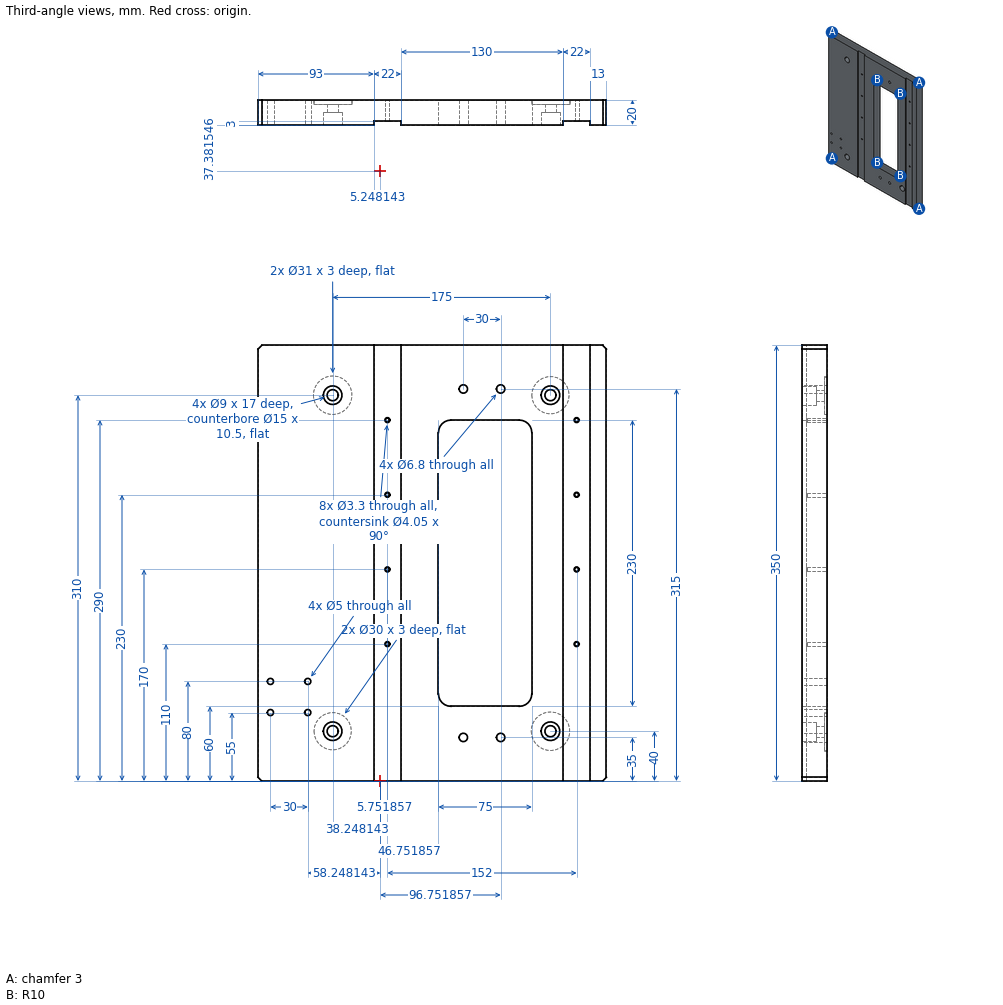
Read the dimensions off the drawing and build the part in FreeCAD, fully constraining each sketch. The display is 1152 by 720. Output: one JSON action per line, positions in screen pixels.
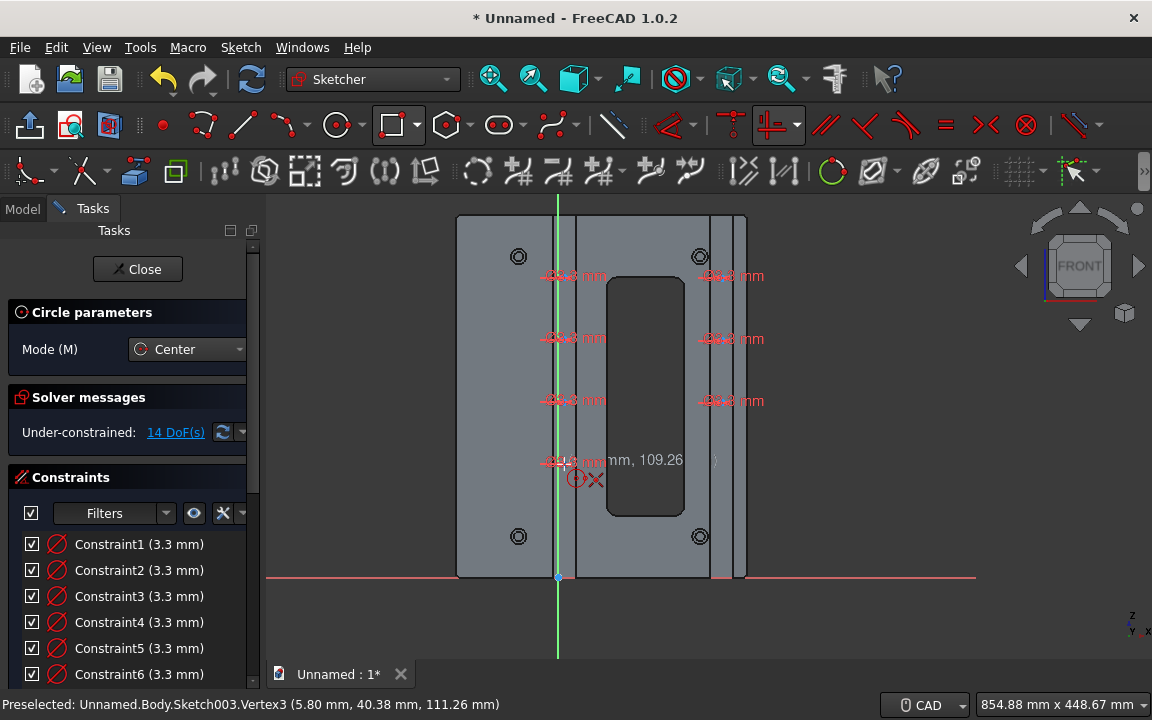
{"action": "scroll", "coordinate": [722, 464], "scroll_direction": "up", "scroll_amount": 13}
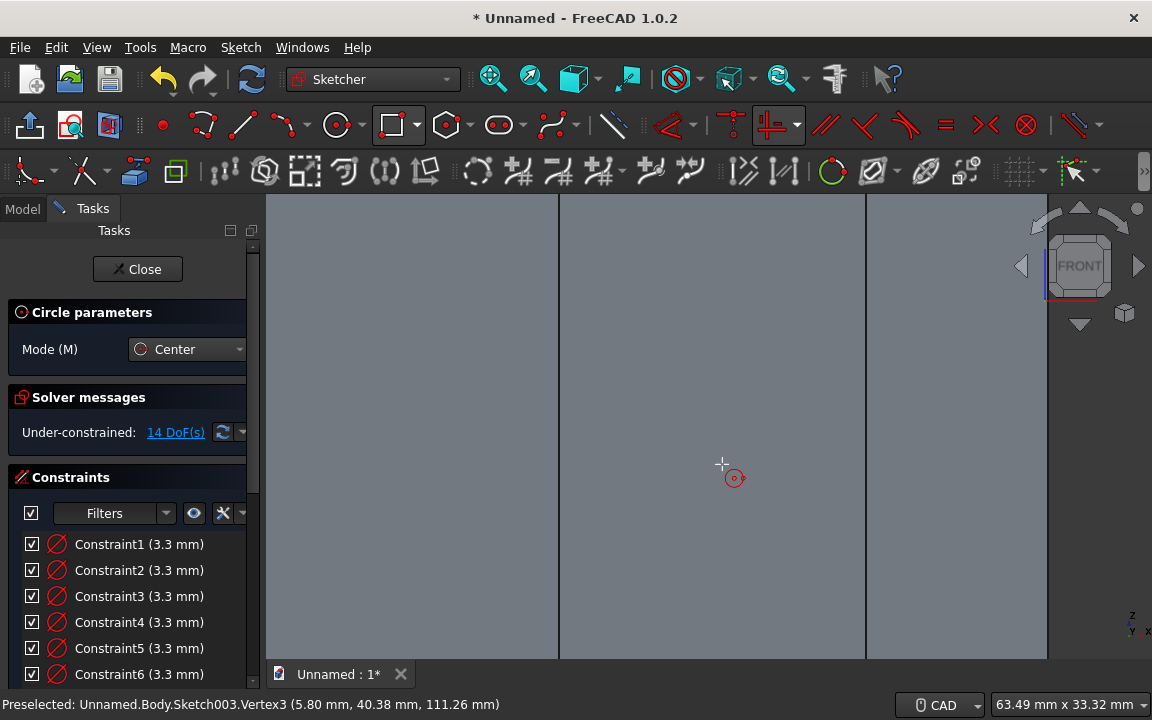
{"action": "scroll", "coordinate": [722, 464], "scroll_direction": "down", "scroll_amount": 13}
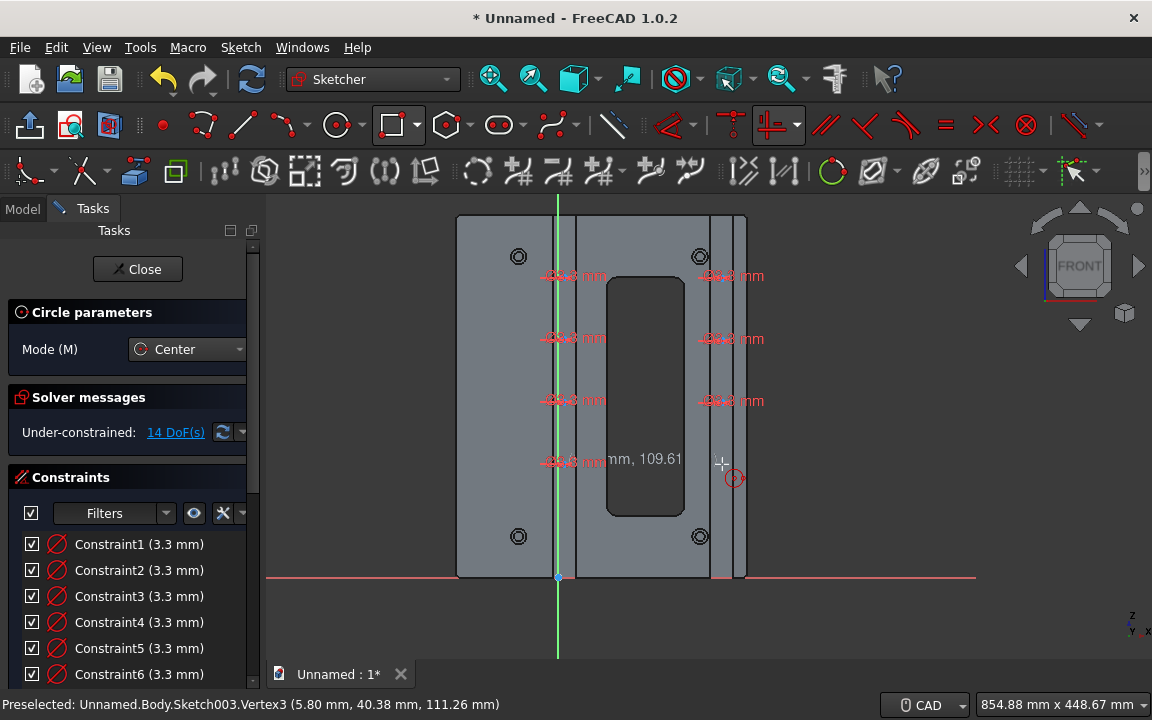
{"action": "left_click", "coordinate": [722, 464]}
{"action": "mouse_move", "coordinate": [723, 463]}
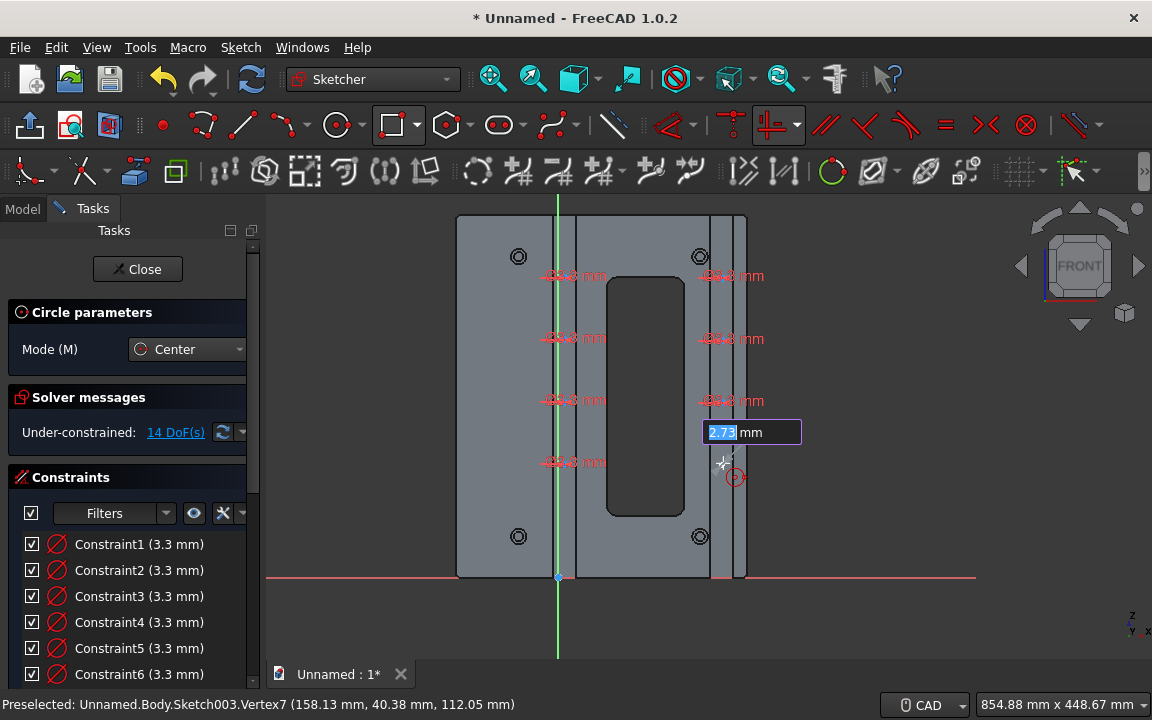
{"action": "type", "text": "3.3"}
{"action": "key", "text": "Return"}
{"action": "key", "text": "Escape"}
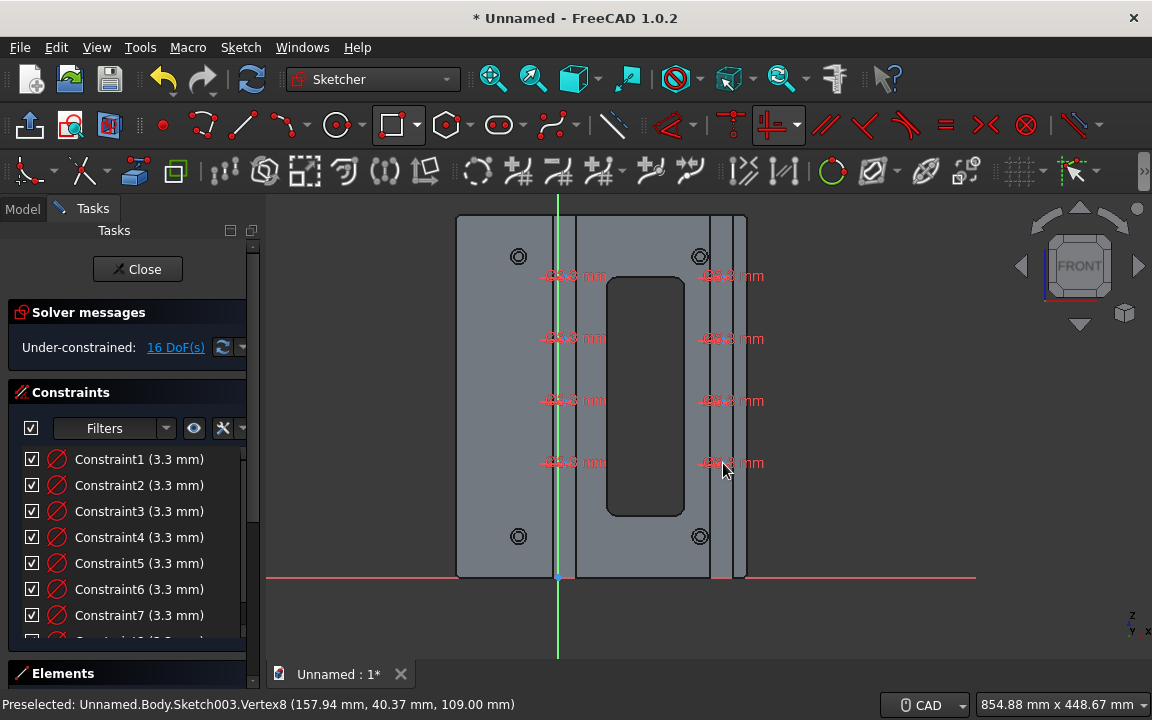
{"action": "left_click", "coordinate": [564, 278]}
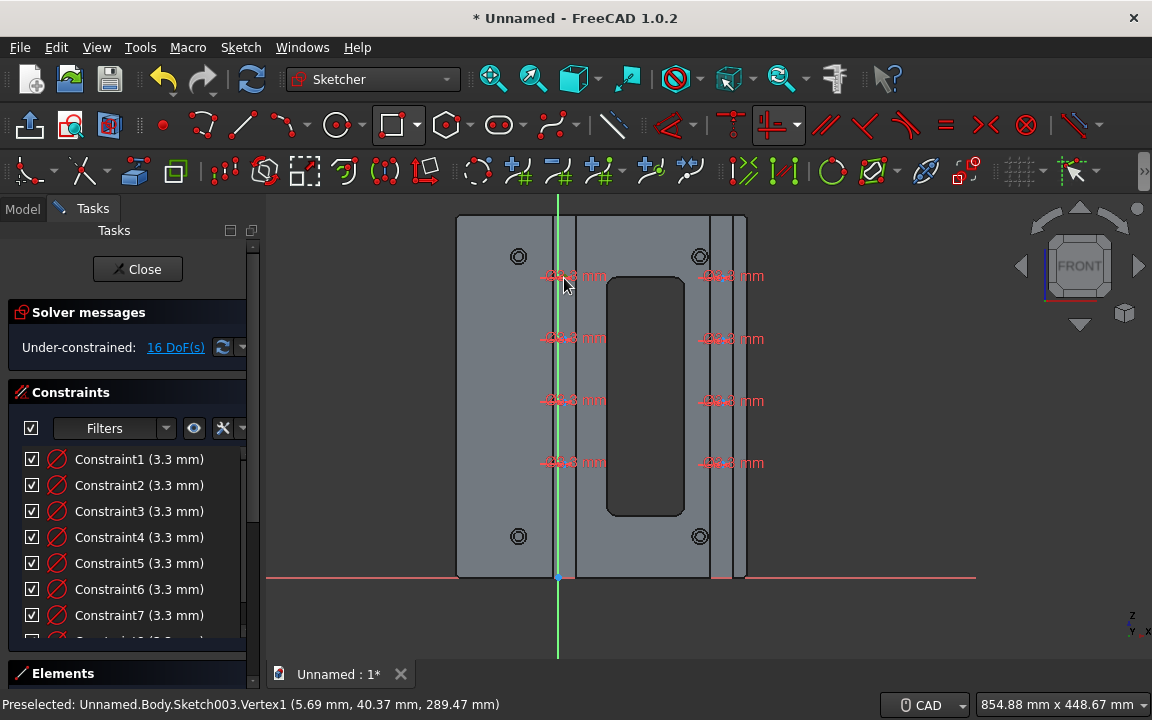
{"action": "left_click", "coordinate": [564, 340]}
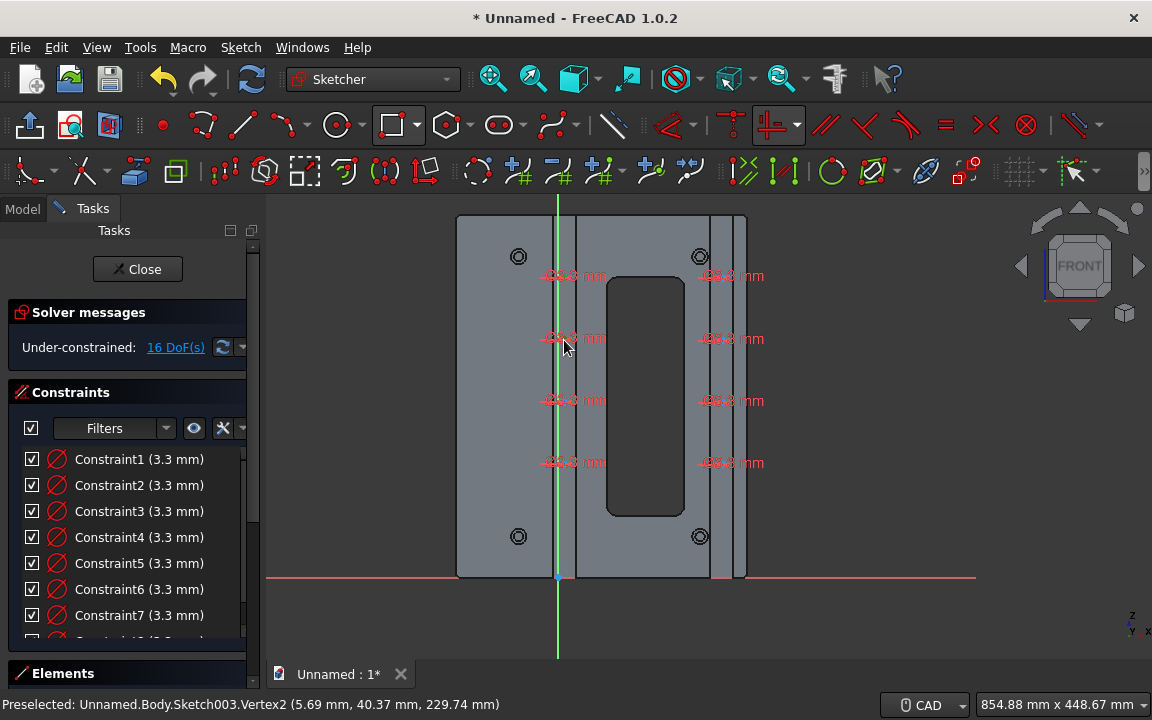
{"action": "key", "text": "v"}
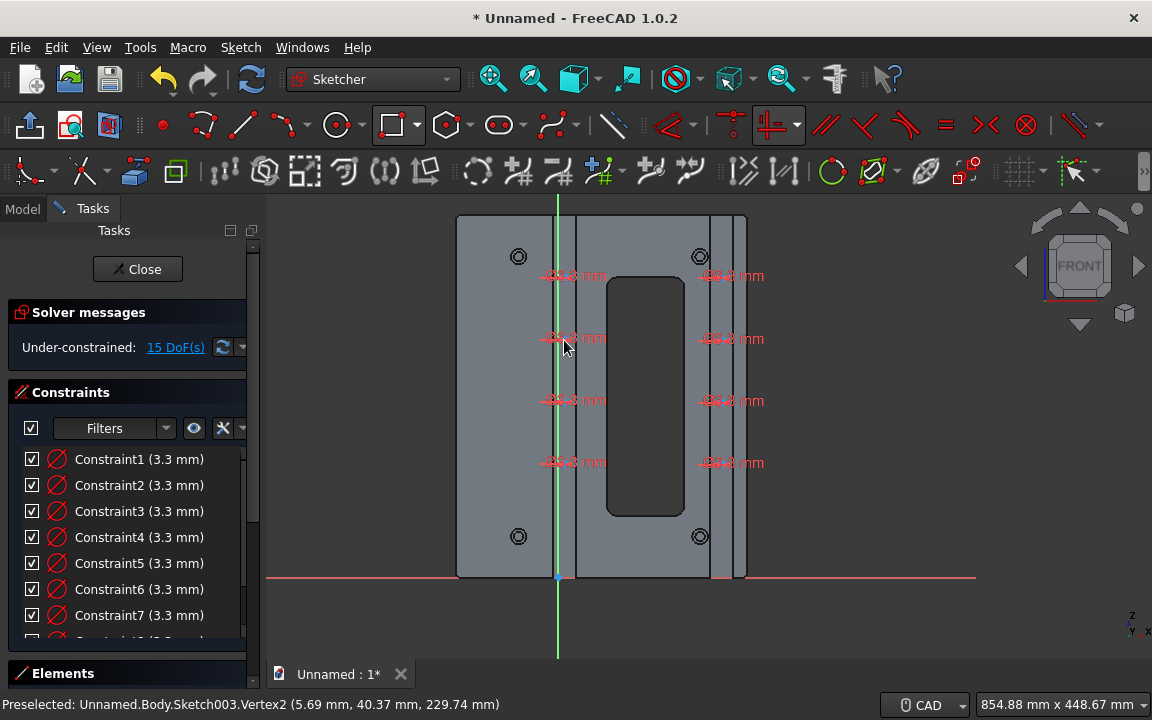
{"action": "left_click", "coordinate": [564, 340]}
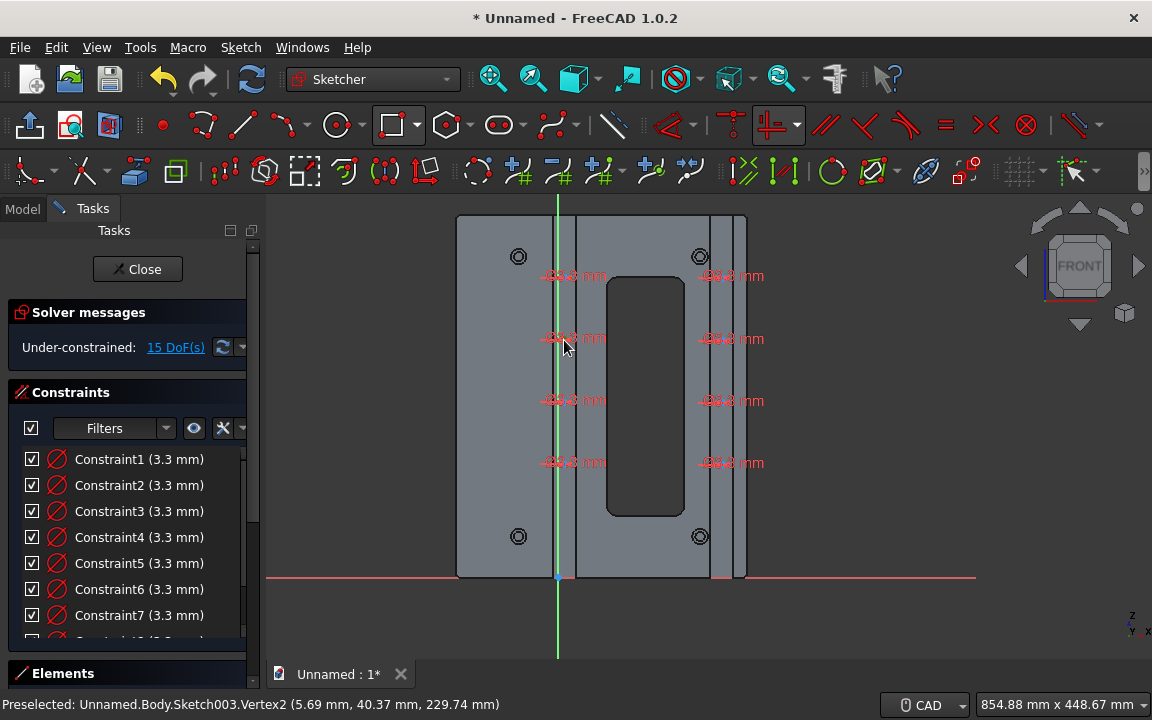
{"action": "left_click", "coordinate": [564, 402]}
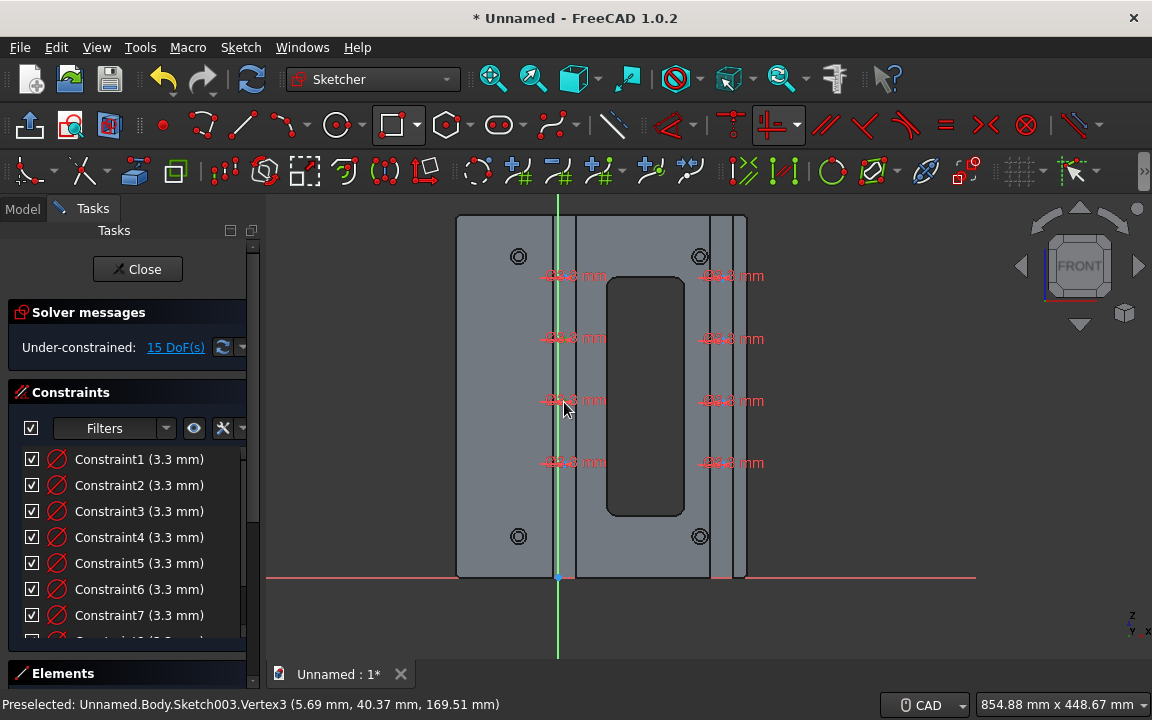
{"action": "left_click", "coordinate": [800, 126]}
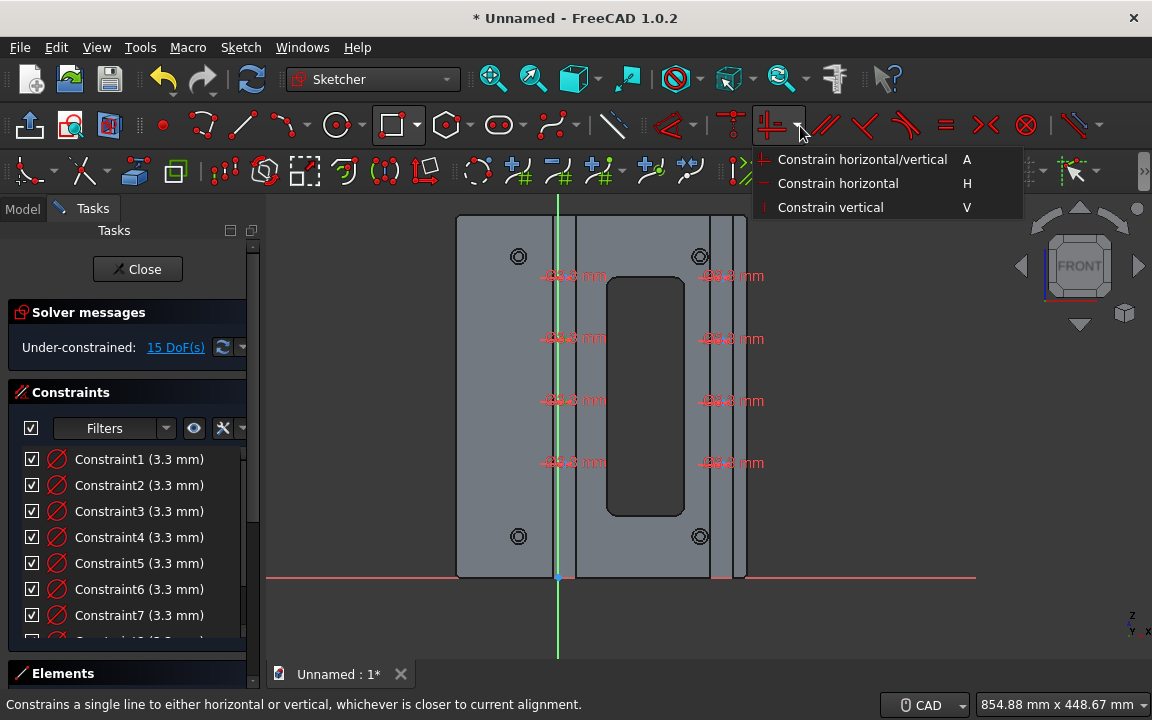
{"action": "left_click", "coordinate": [888, 207]}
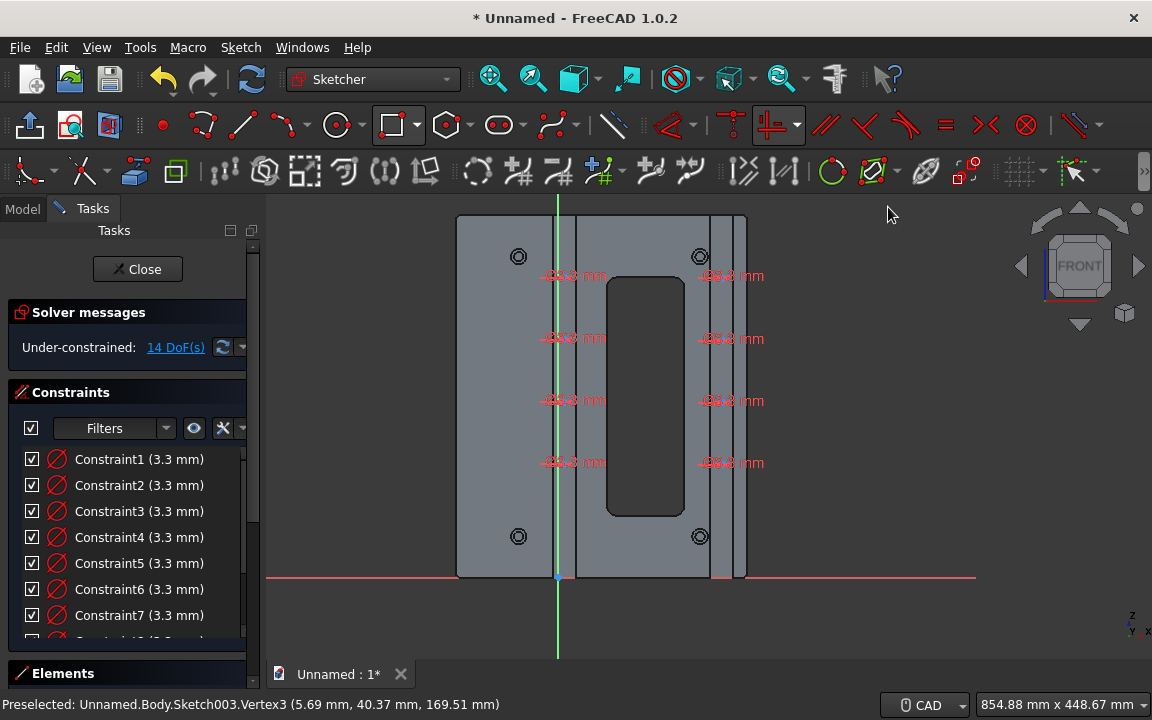
{"action": "left_click", "coordinate": [564, 402]}